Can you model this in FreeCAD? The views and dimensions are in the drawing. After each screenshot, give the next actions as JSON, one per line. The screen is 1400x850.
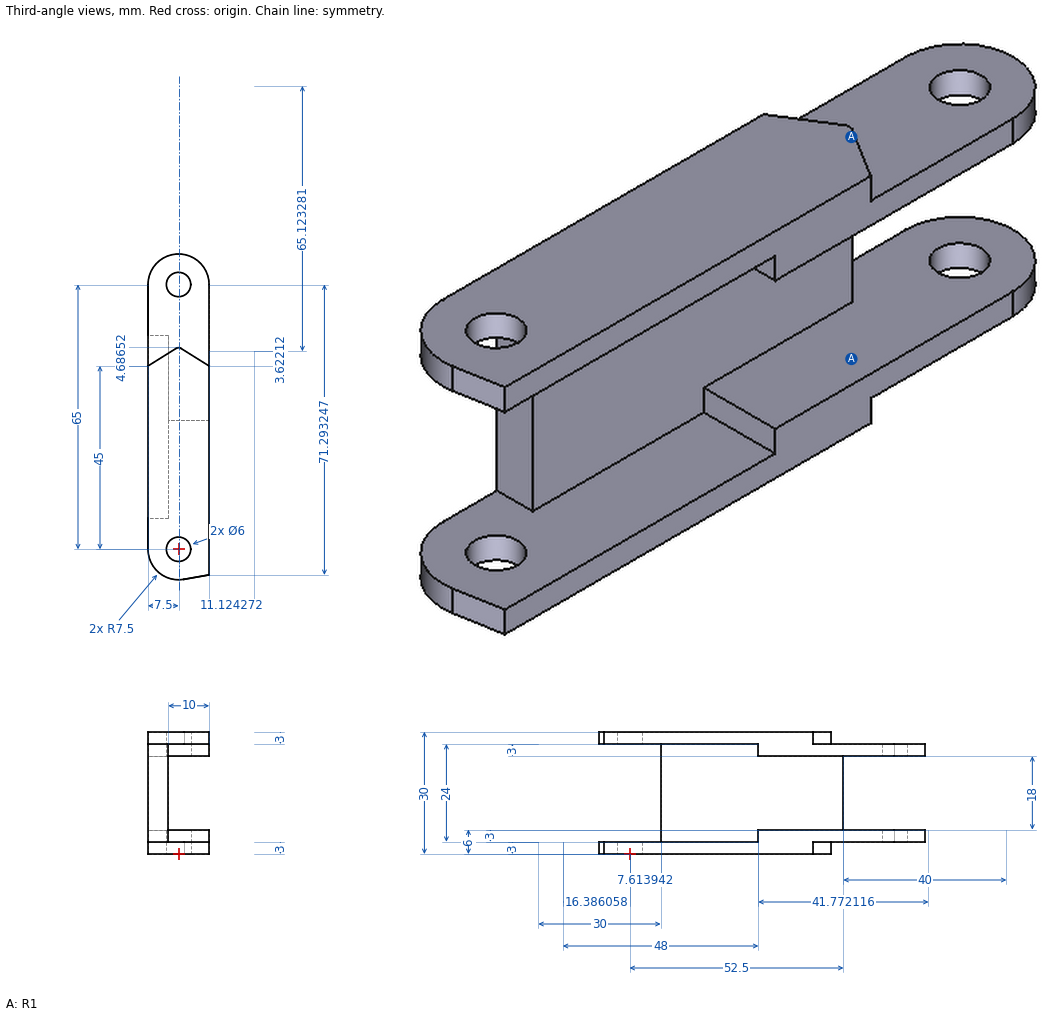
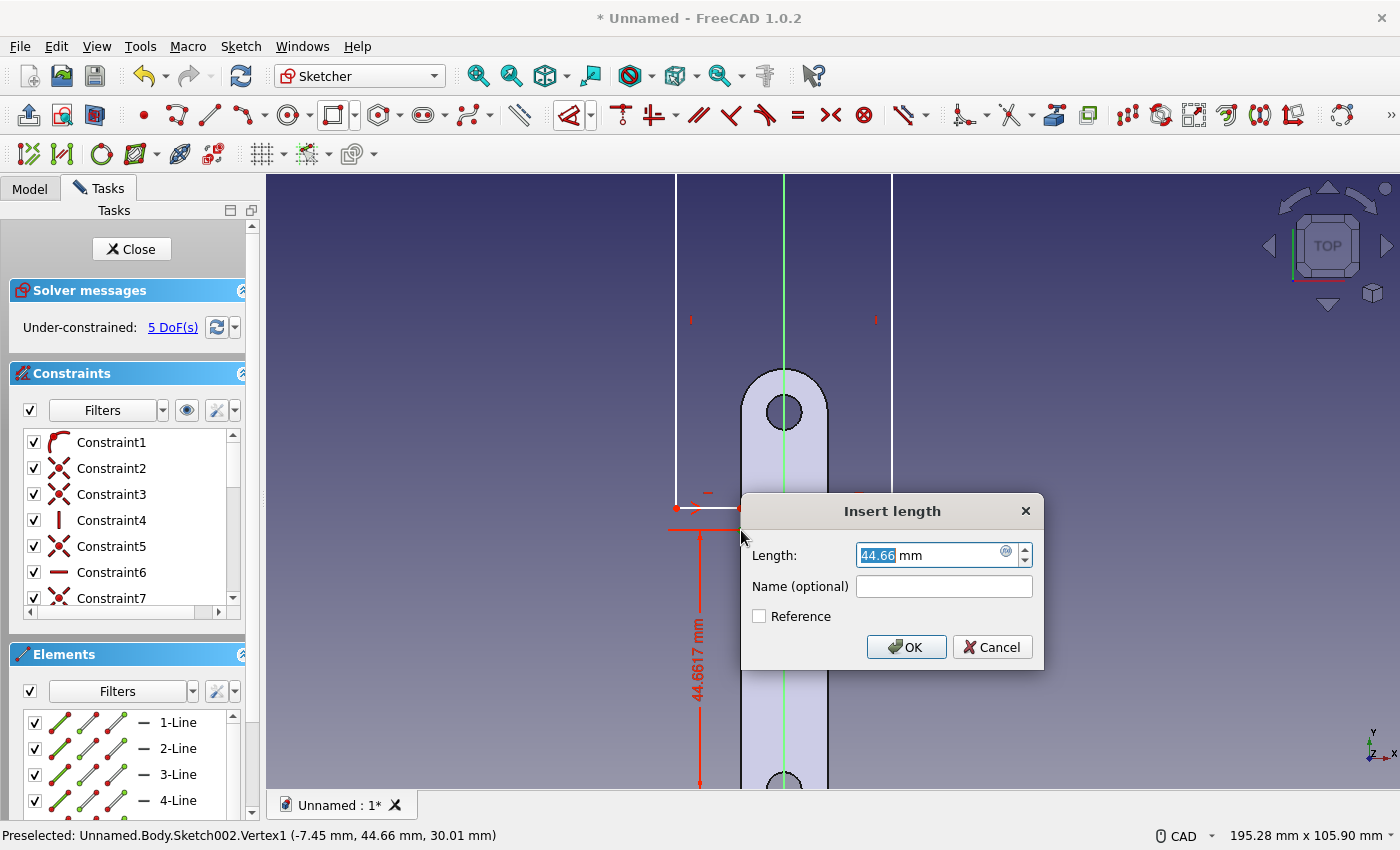
{"action": "type", "text": "45"}
{"action": "key", "text": "Return"}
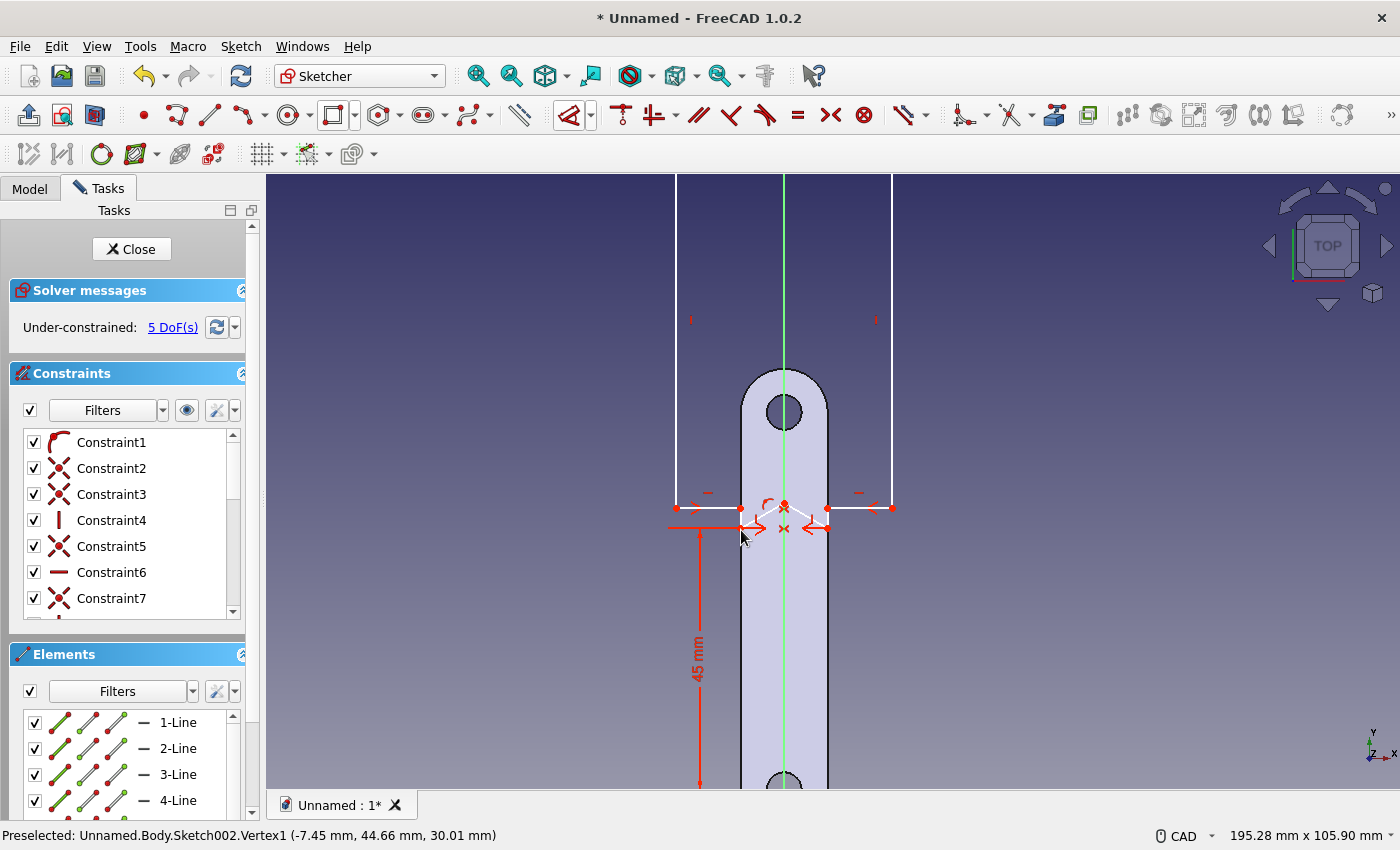
{"action": "left_click", "coordinate": [741, 528]}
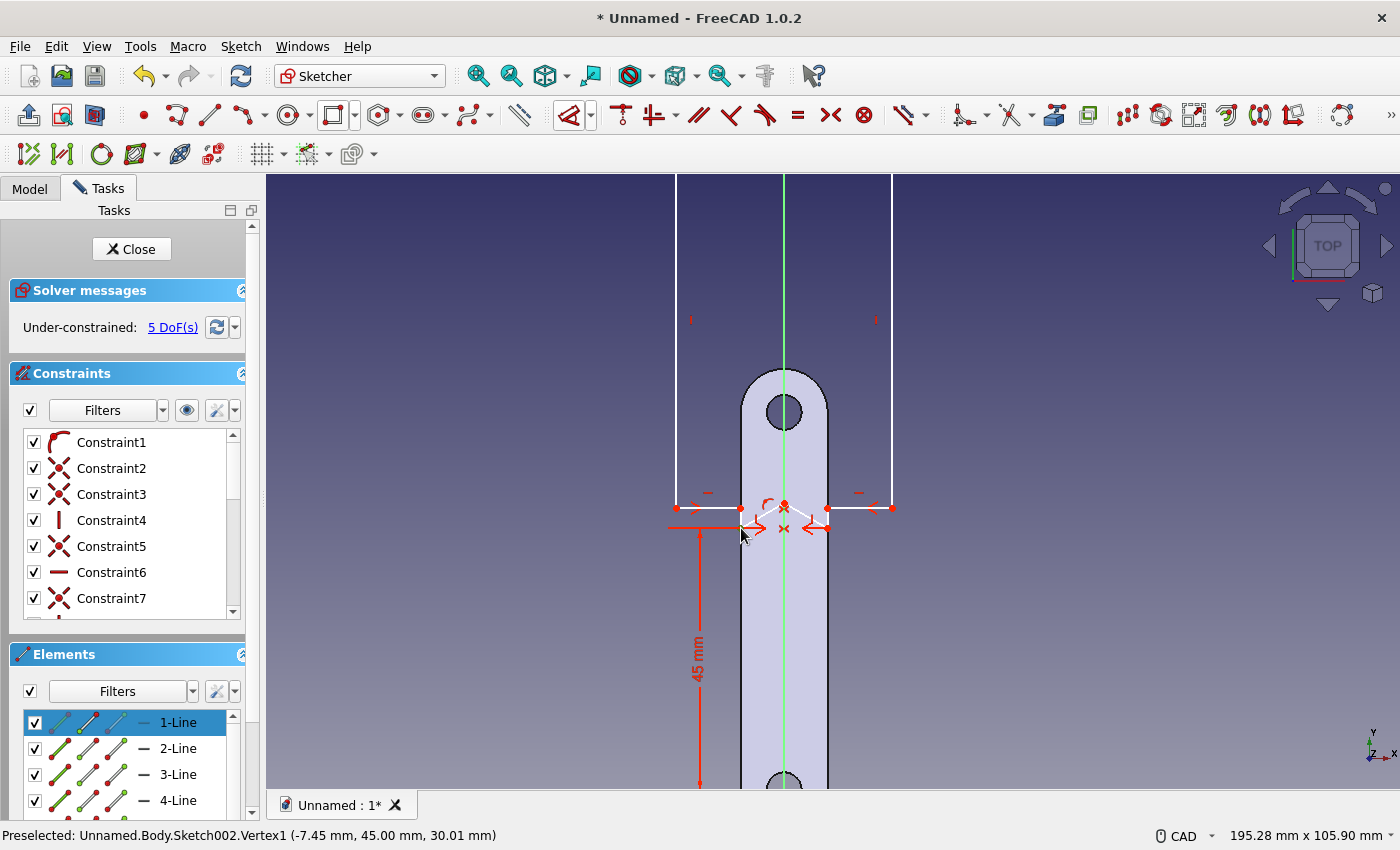
{"action": "key", "text": "l"}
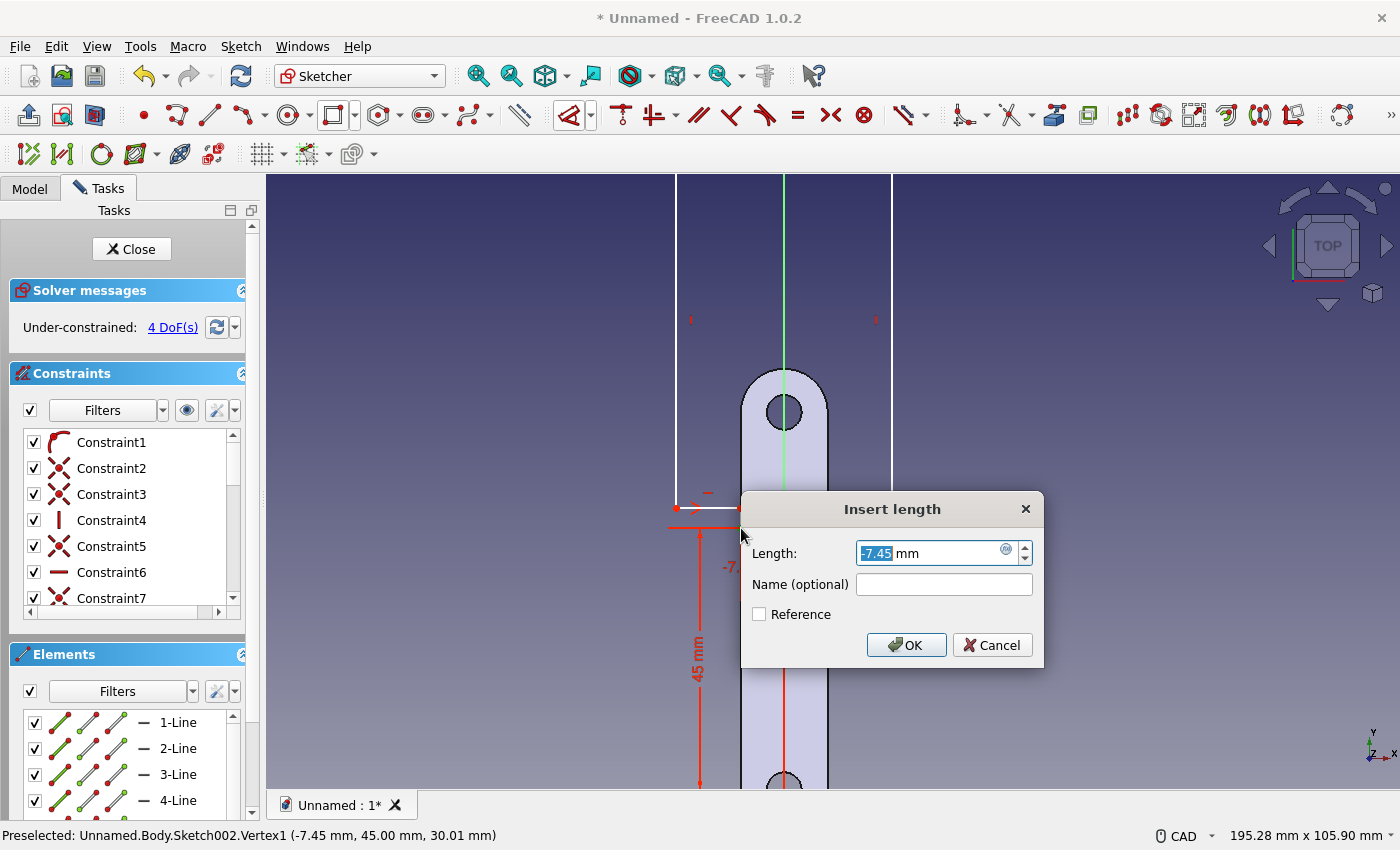
{"action": "type", "text": "-7.5"}
{"action": "key", "text": "Return"}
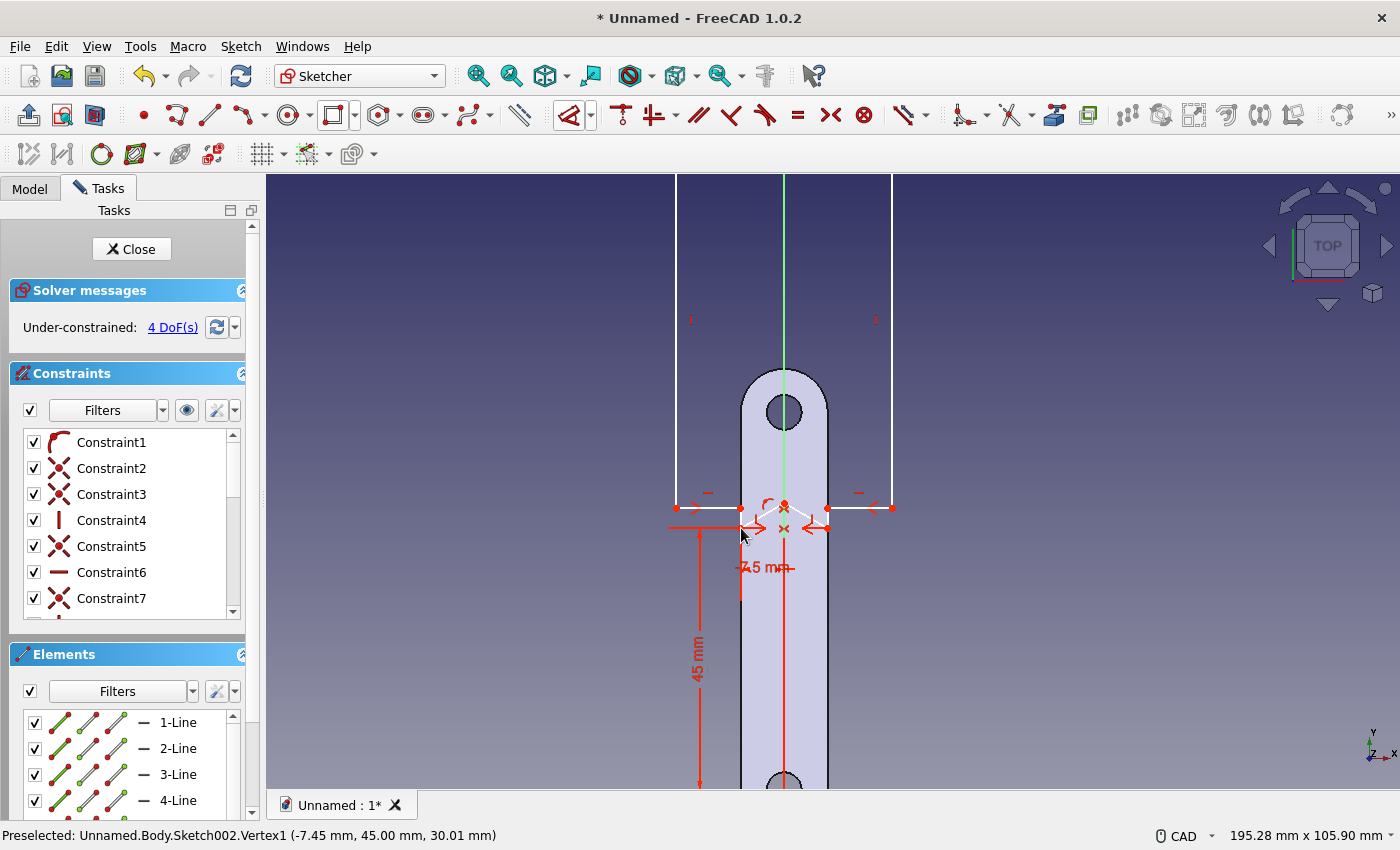
{"action": "scroll", "coordinate": [828, 518], "scroll_direction": "up", "scroll_amount": 4}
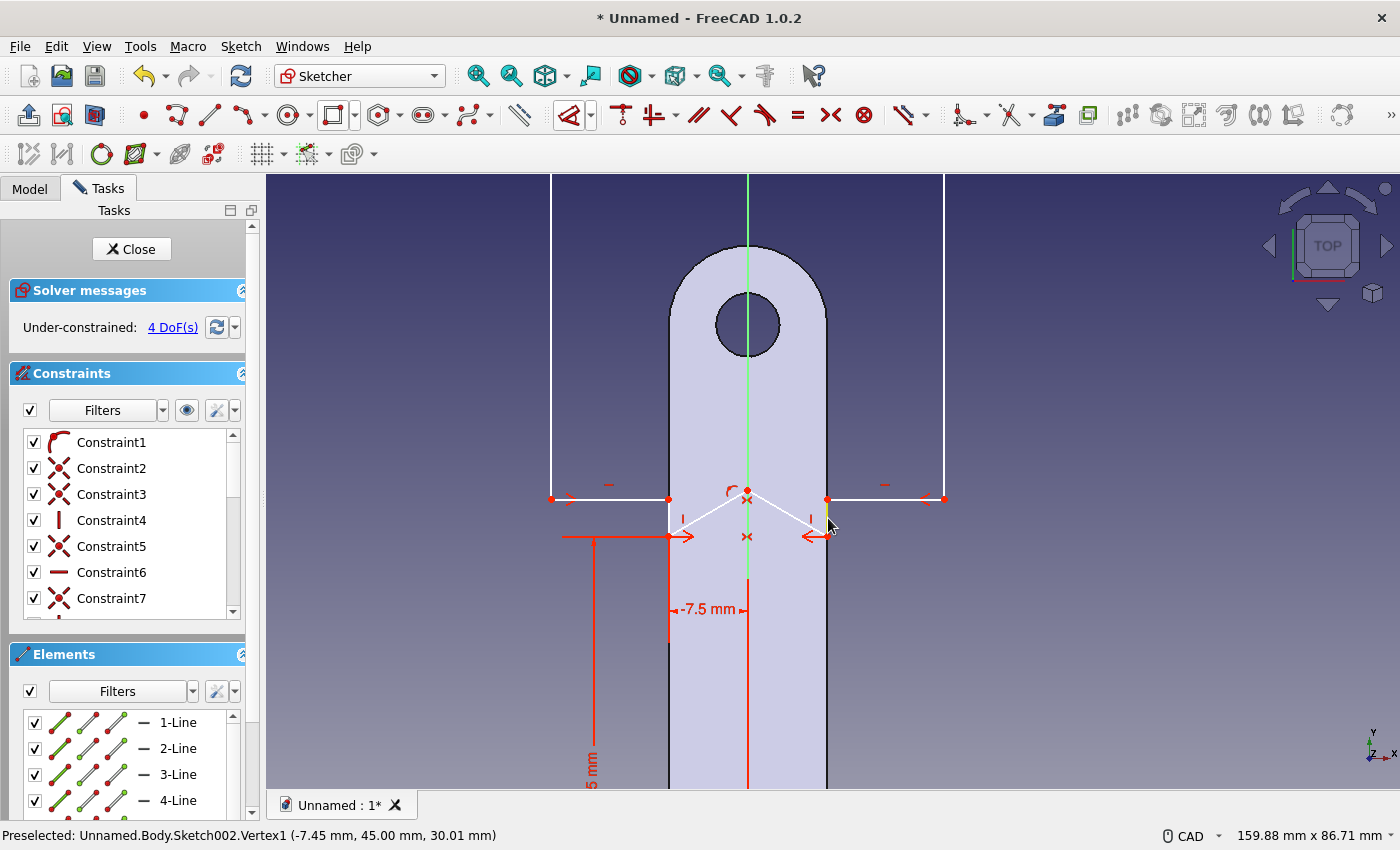
{"action": "left_click", "coordinate": [827, 518]}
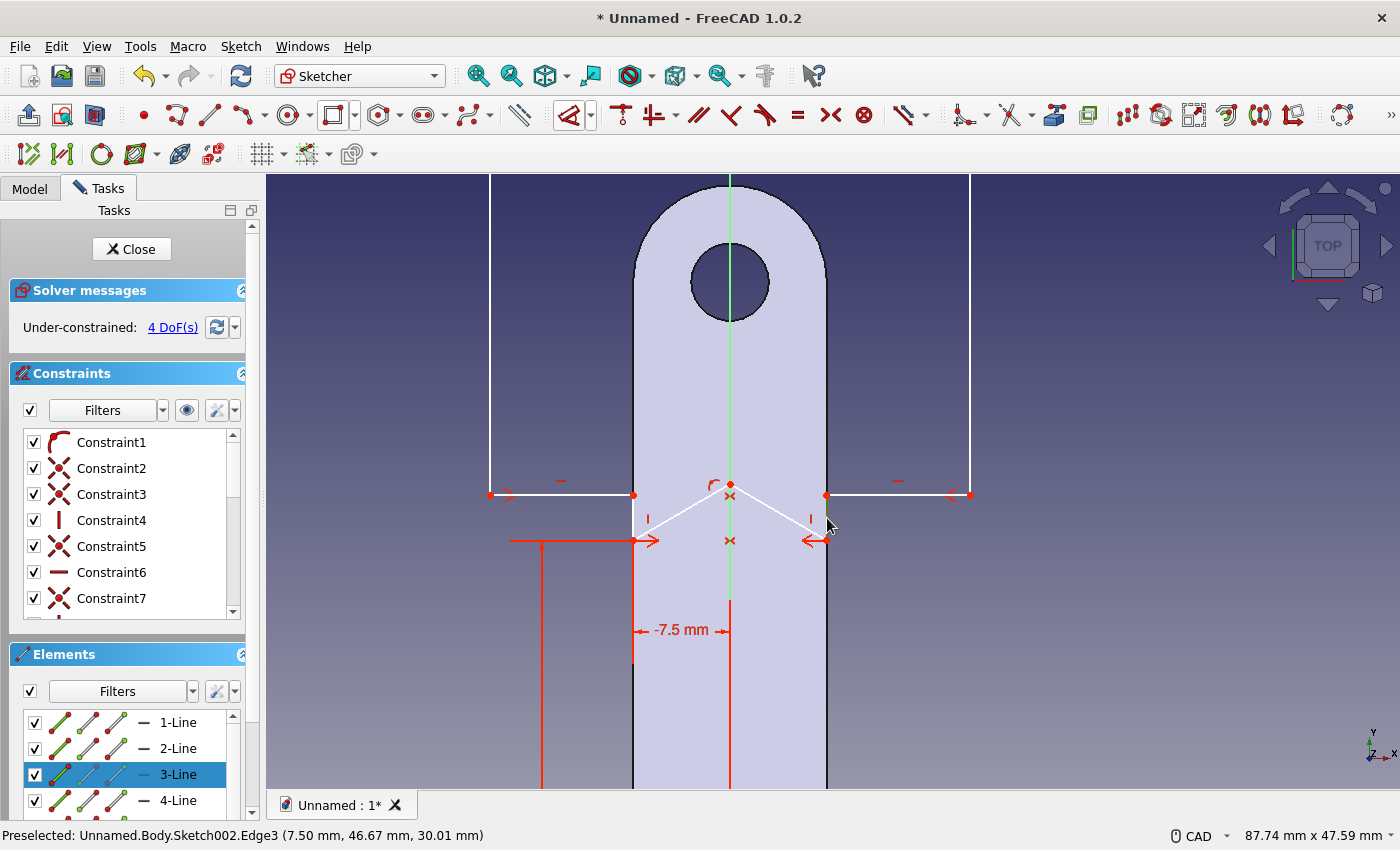
{"action": "key", "text": "i"}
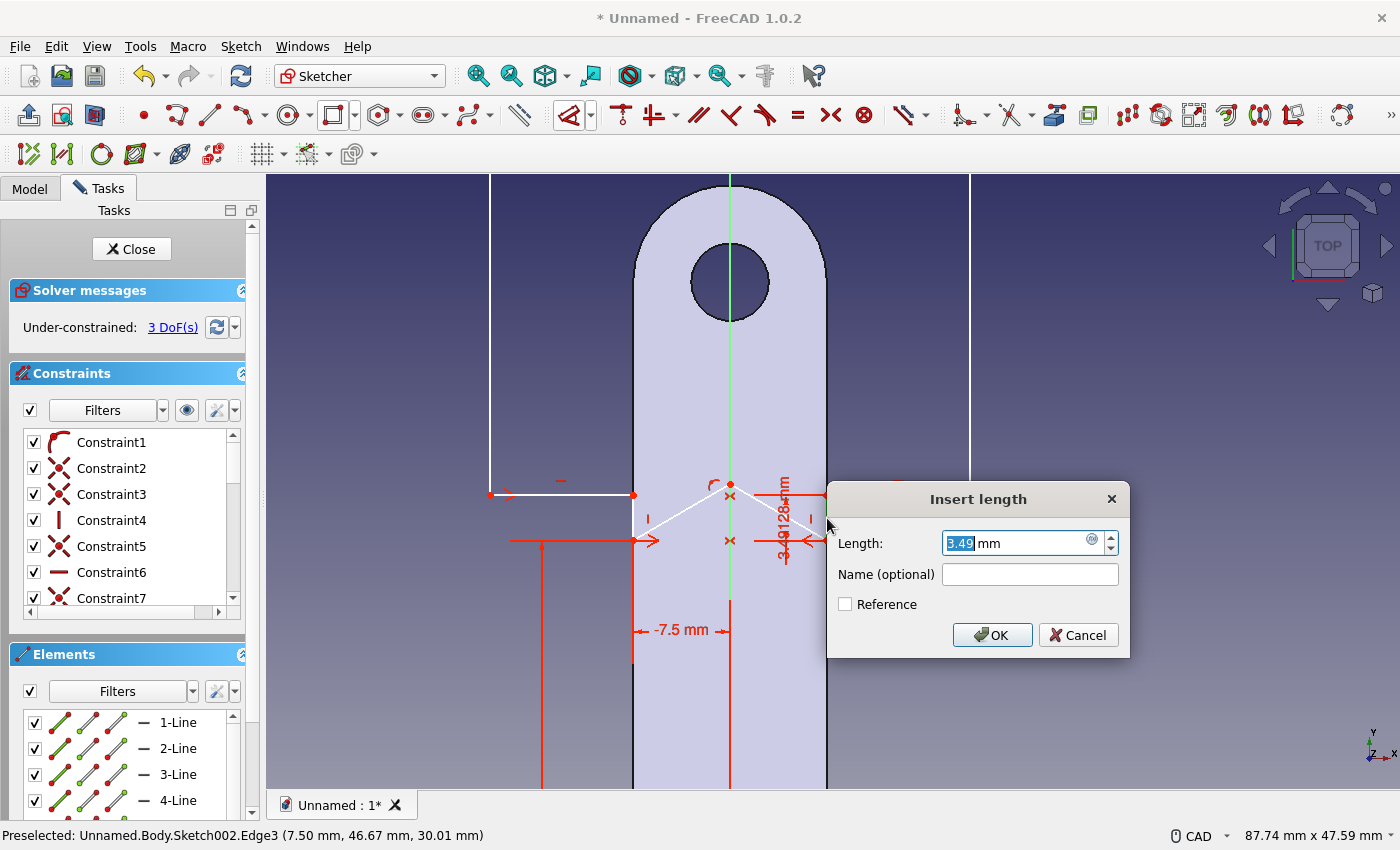
{"action": "type", "text": "3.62212"}
{"action": "key", "text": "Return"}